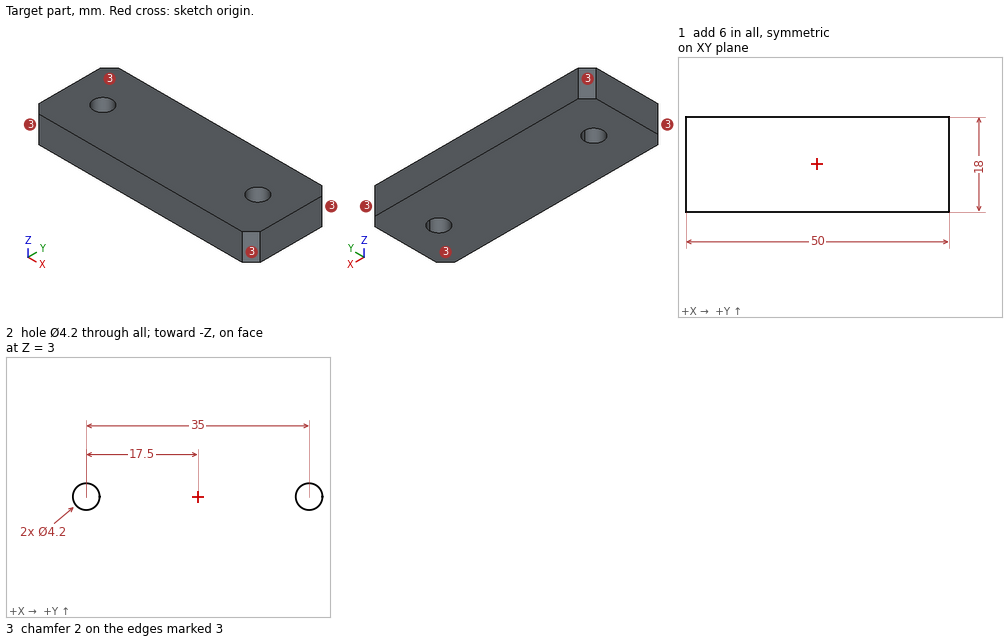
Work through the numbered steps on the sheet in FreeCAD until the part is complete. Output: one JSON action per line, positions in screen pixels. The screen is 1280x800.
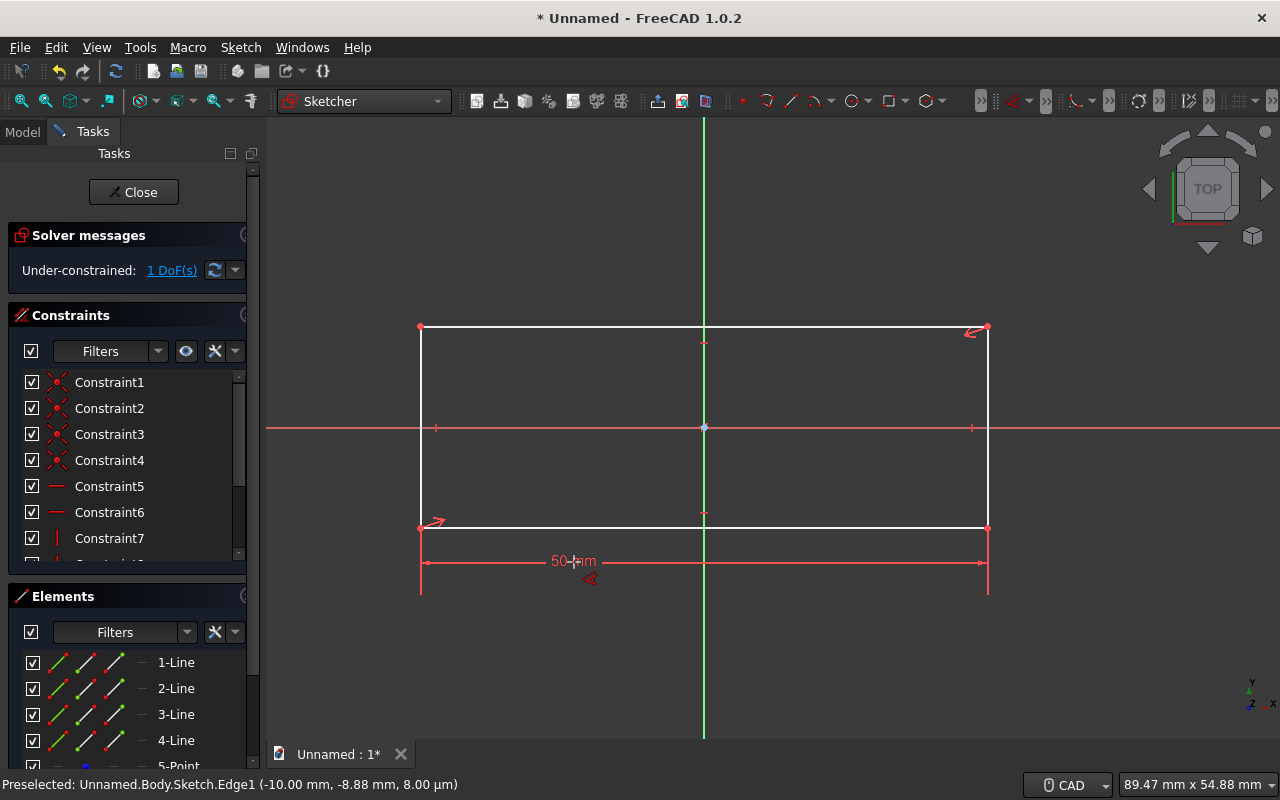
{"action": "left_click", "coordinate": [988, 468]}
{"action": "left_click", "coordinate": [1022, 381]}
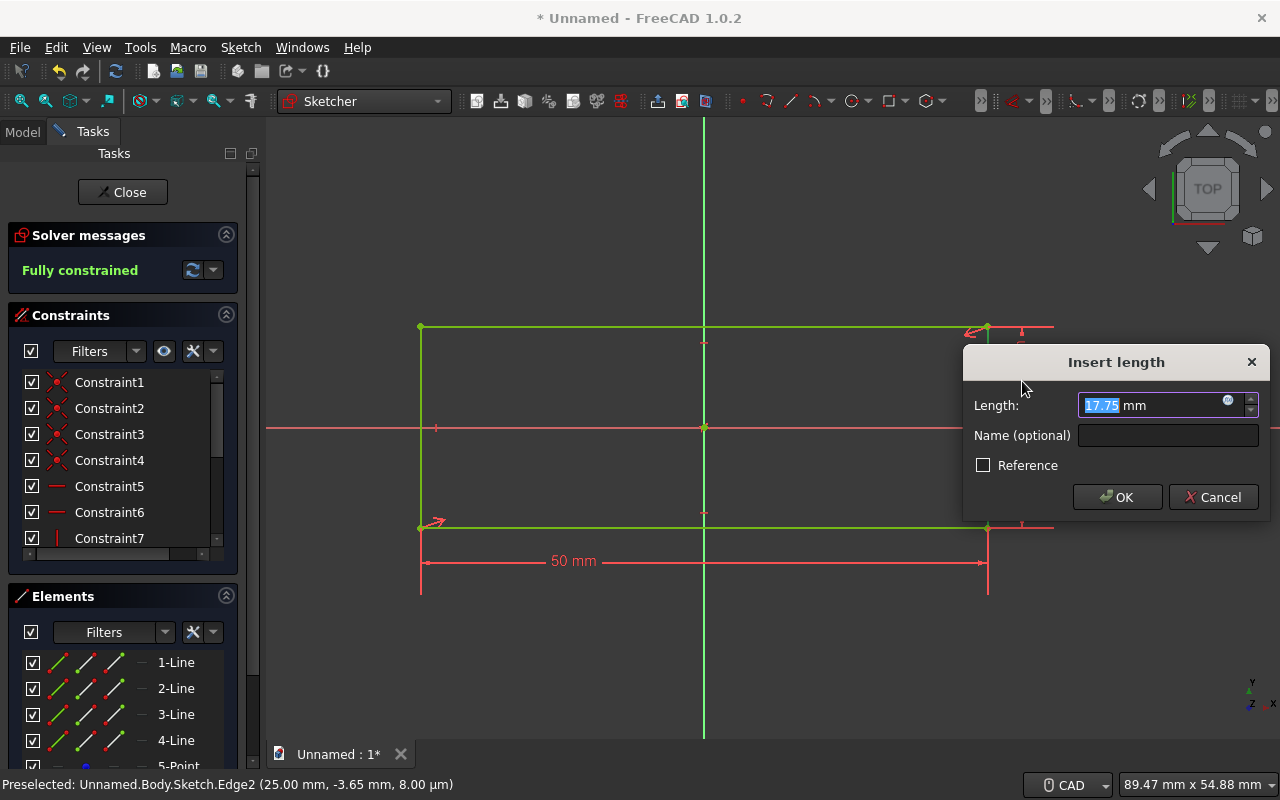
{"action": "type", "text": "18"}
{"action": "key", "text": "Return"}
{"action": "key", "text": "Escape"}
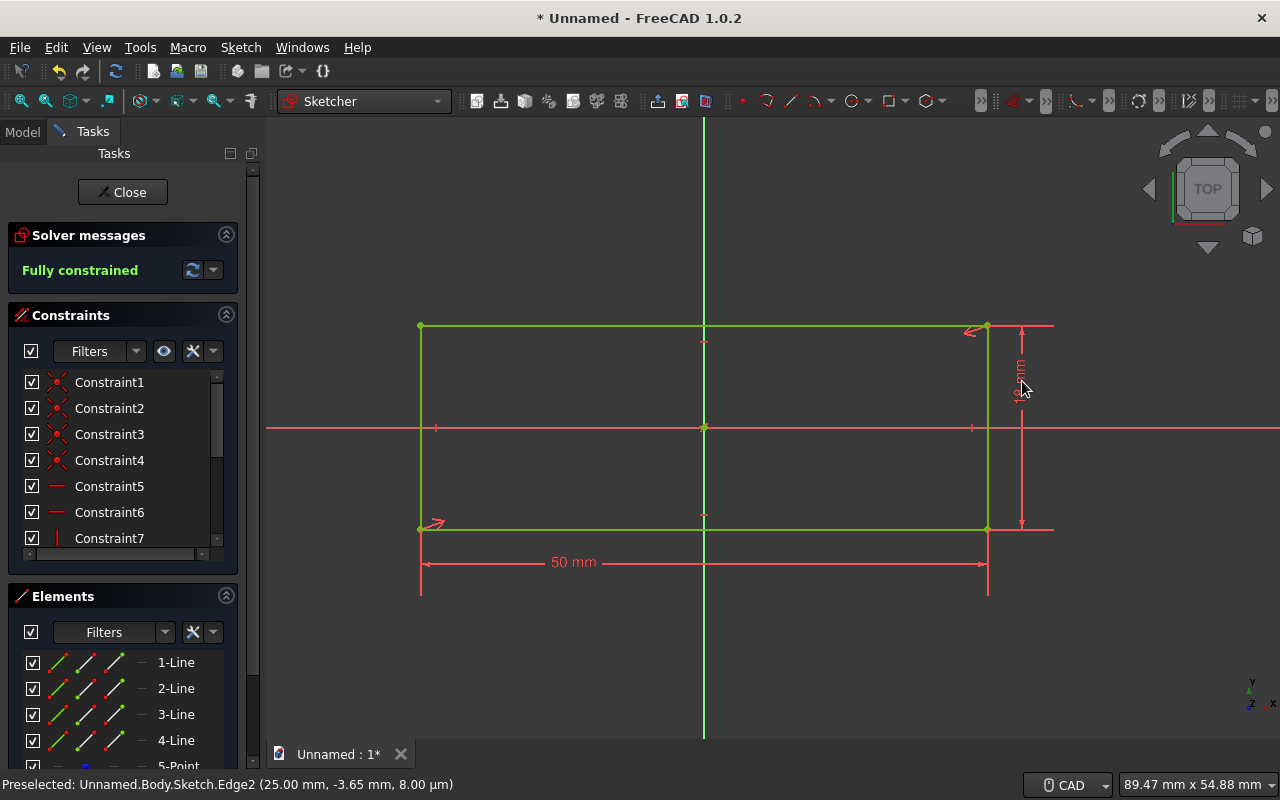
{"action": "left_click", "coordinate": [123, 192]}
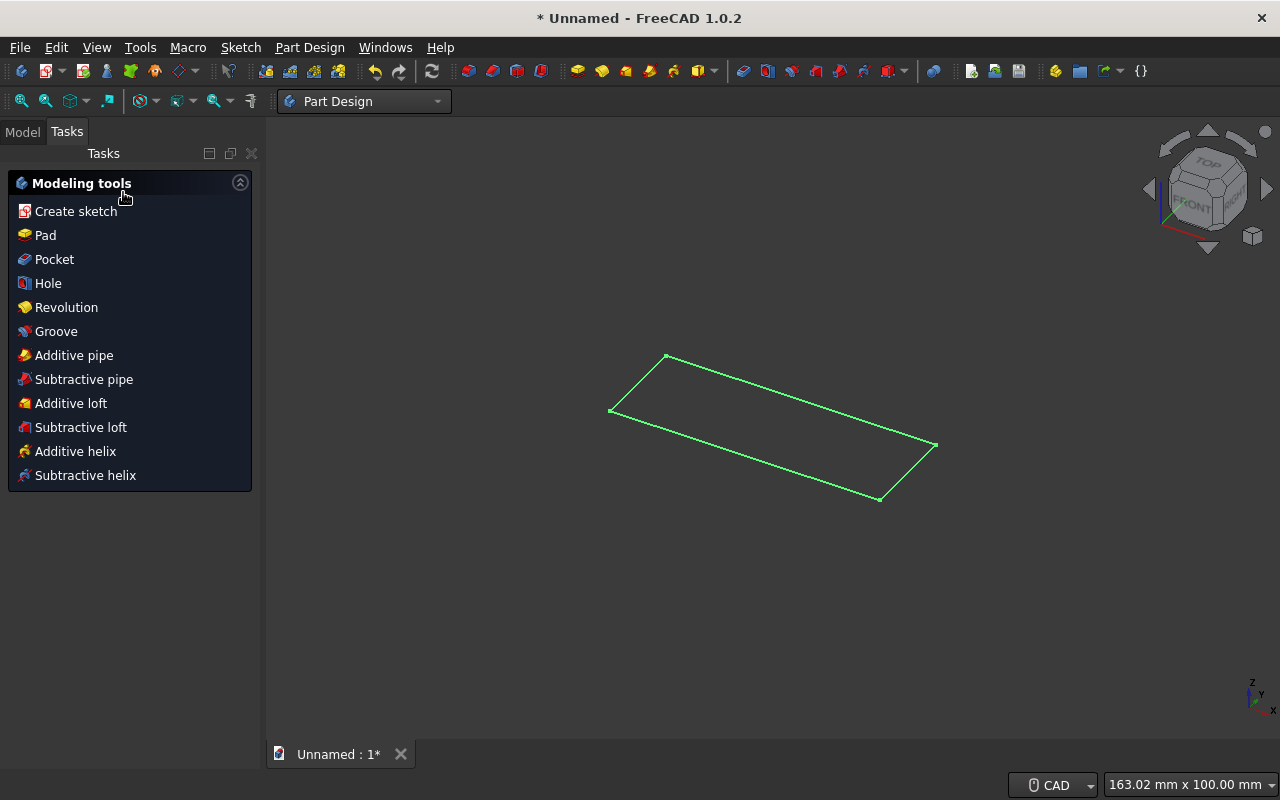
{"action": "left_click", "coordinate": [578, 72]}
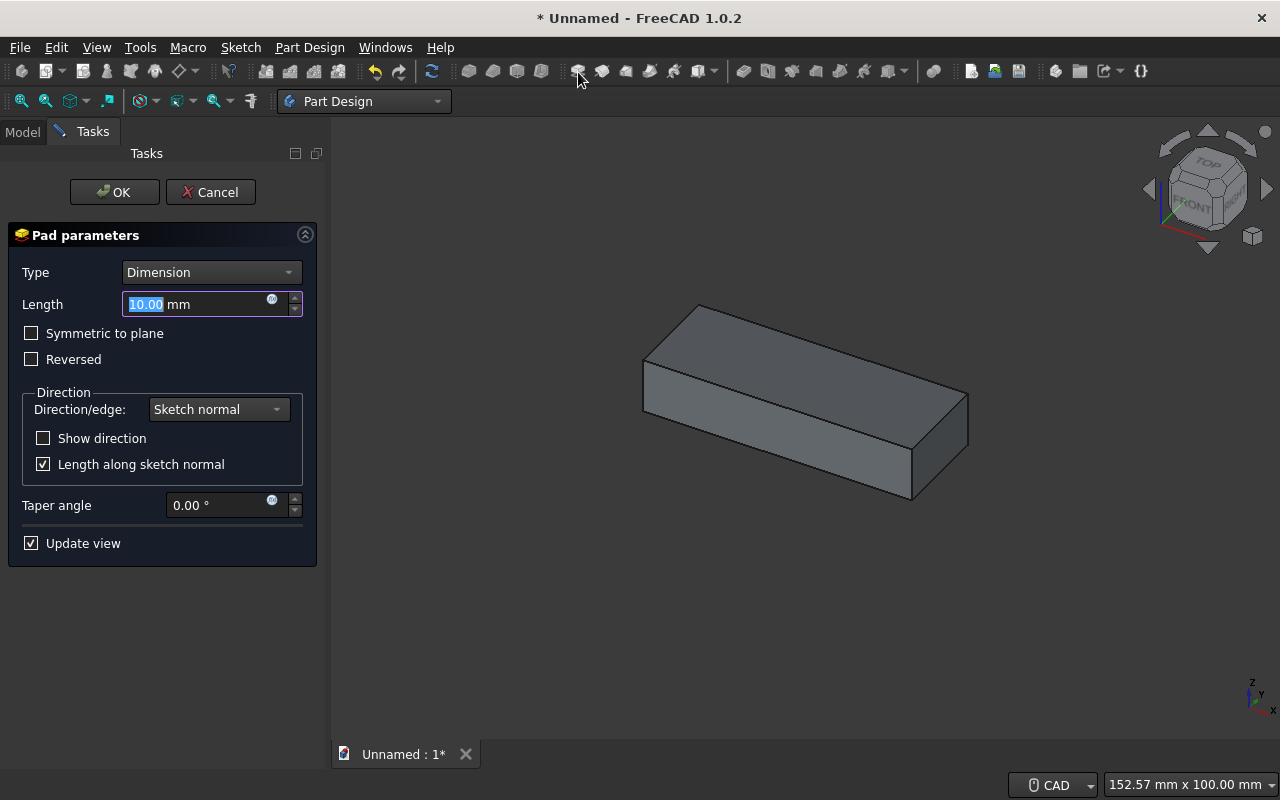
{"action": "type", "text": "6"}
{"action": "key", "text": "Tab"}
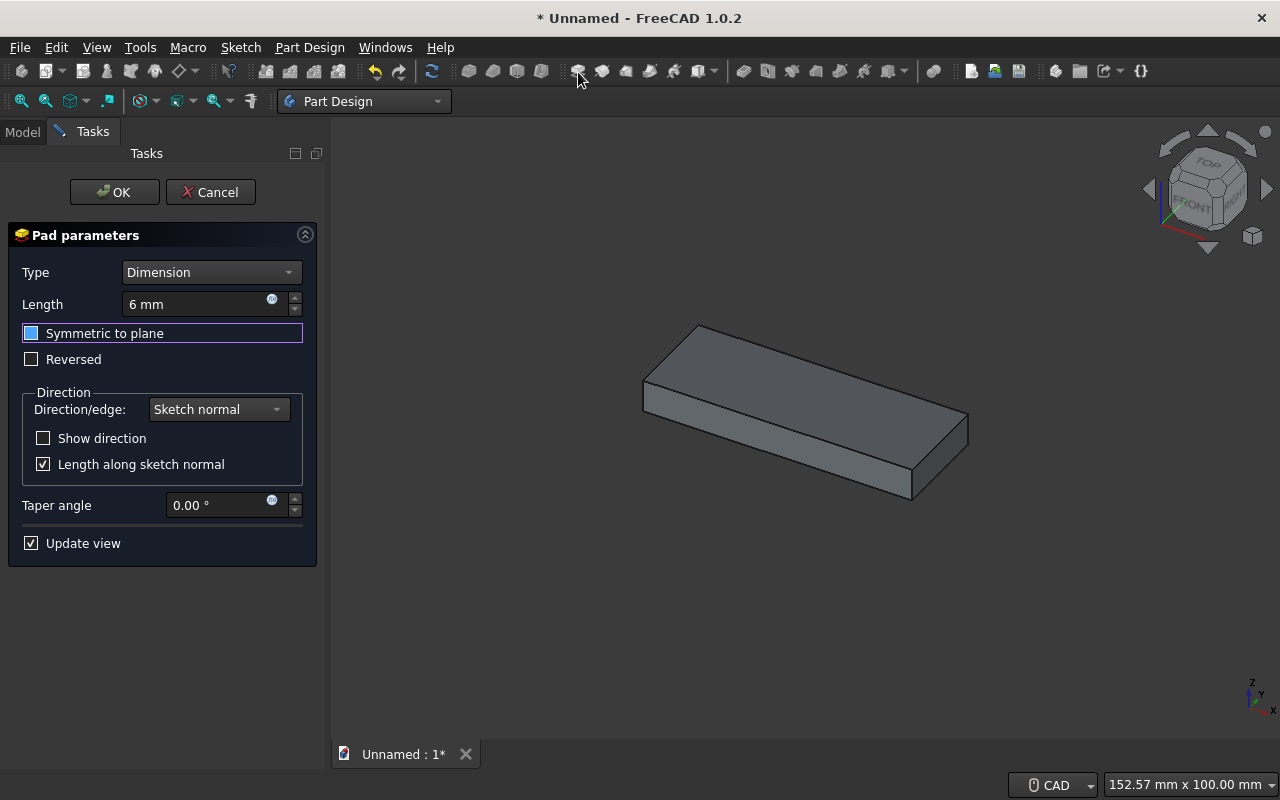
{"action": "left_click", "coordinate": [30, 333]}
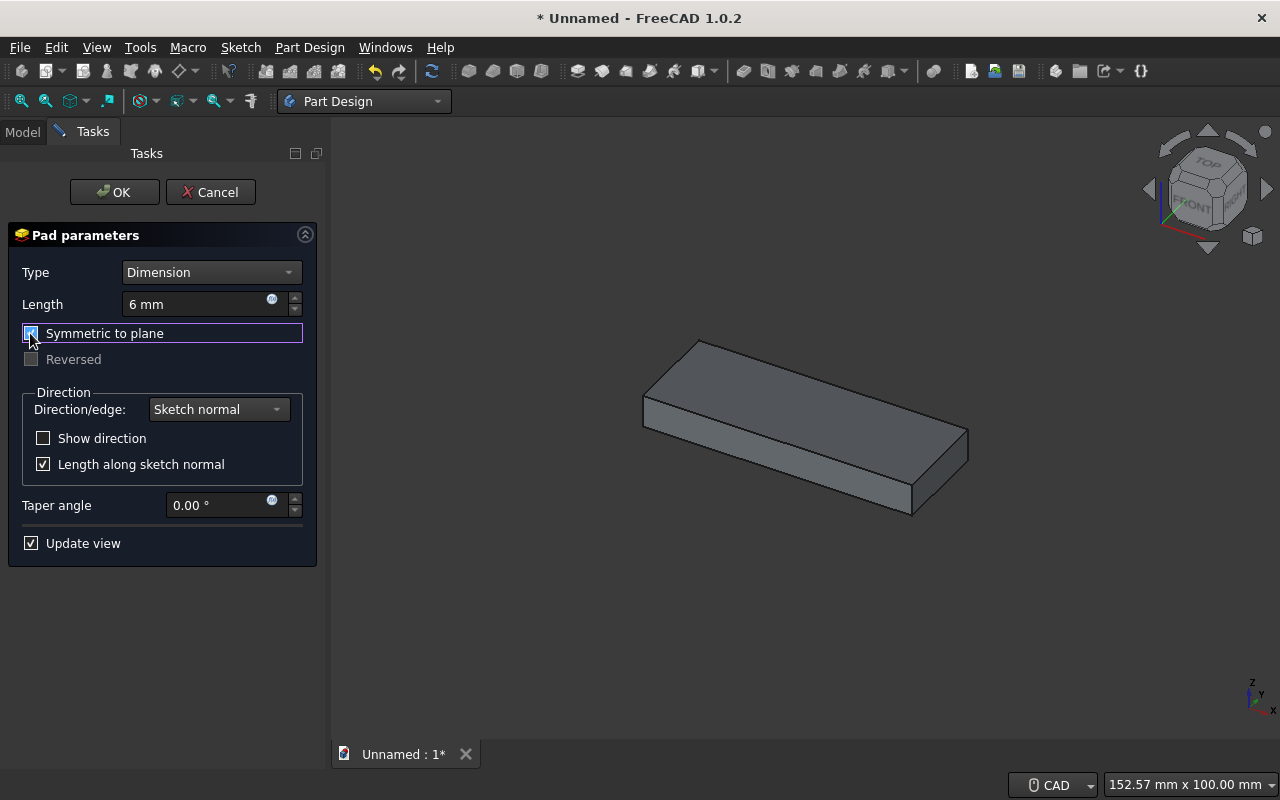
{"action": "left_click", "coordinate": [115, 192]}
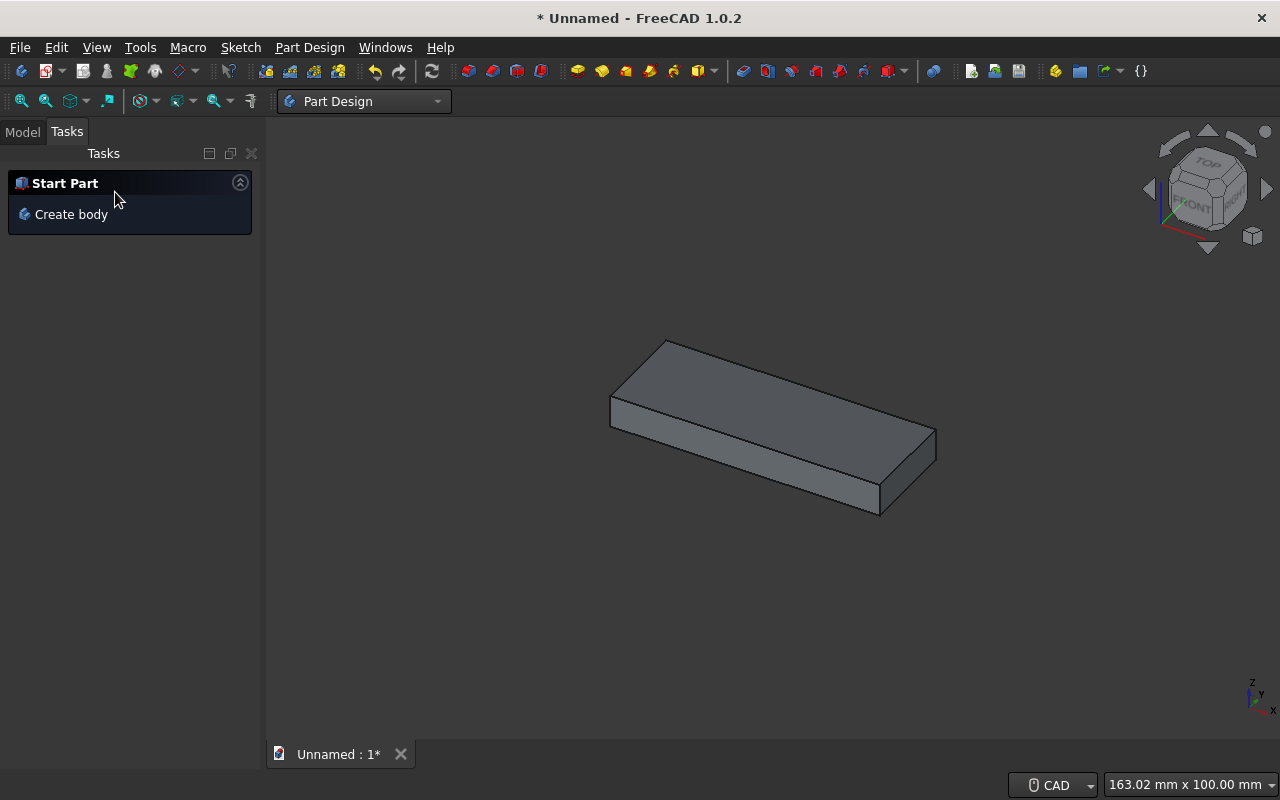
{"action": "key", "text": "v f"}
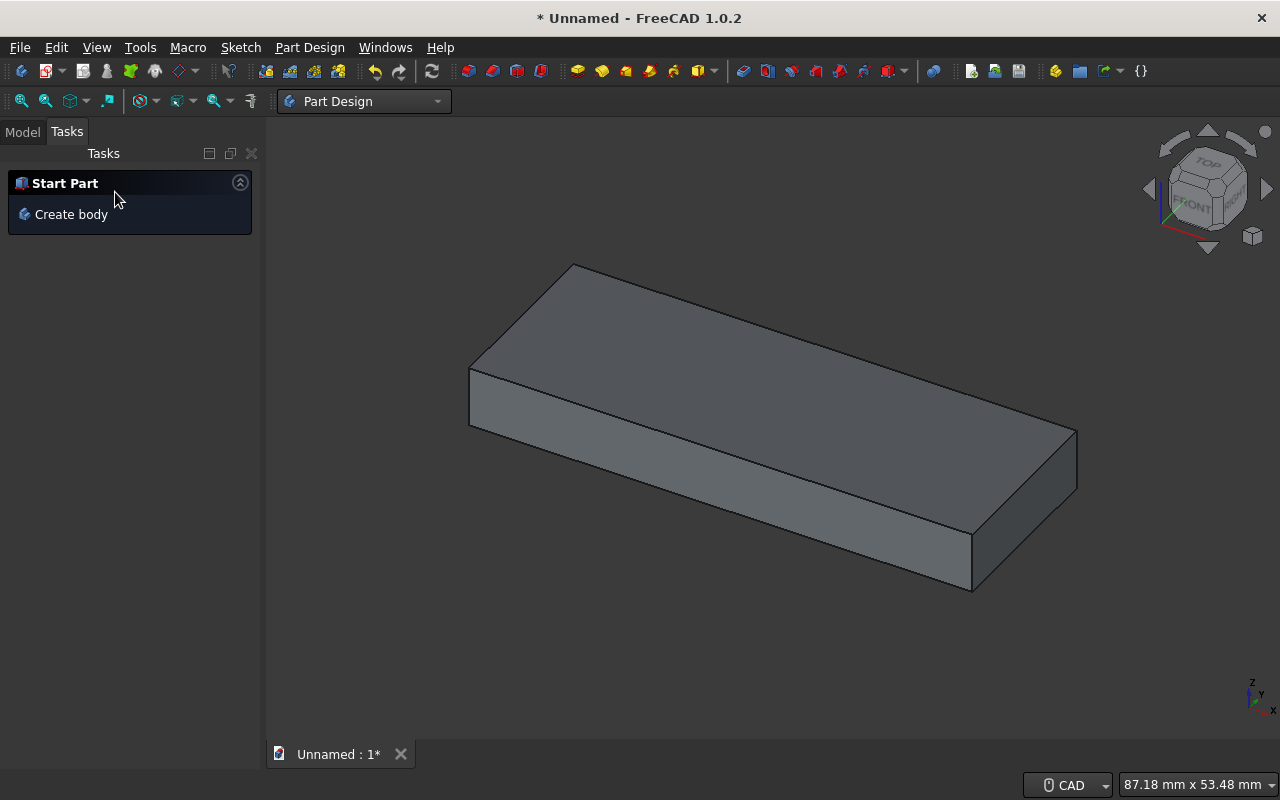
{"action": "left_click", "coordinate": [917, 446]}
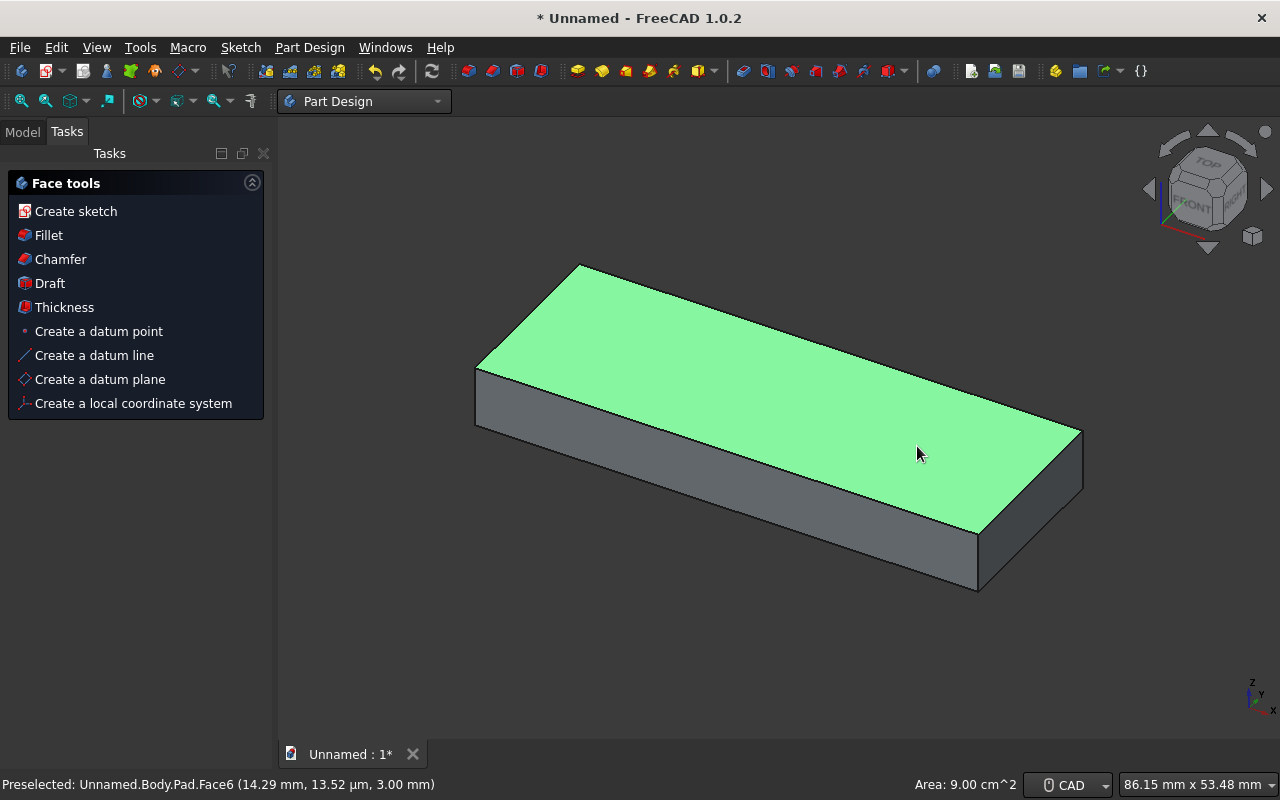
{"action": "left_click", "coordinate": [46, 72]}